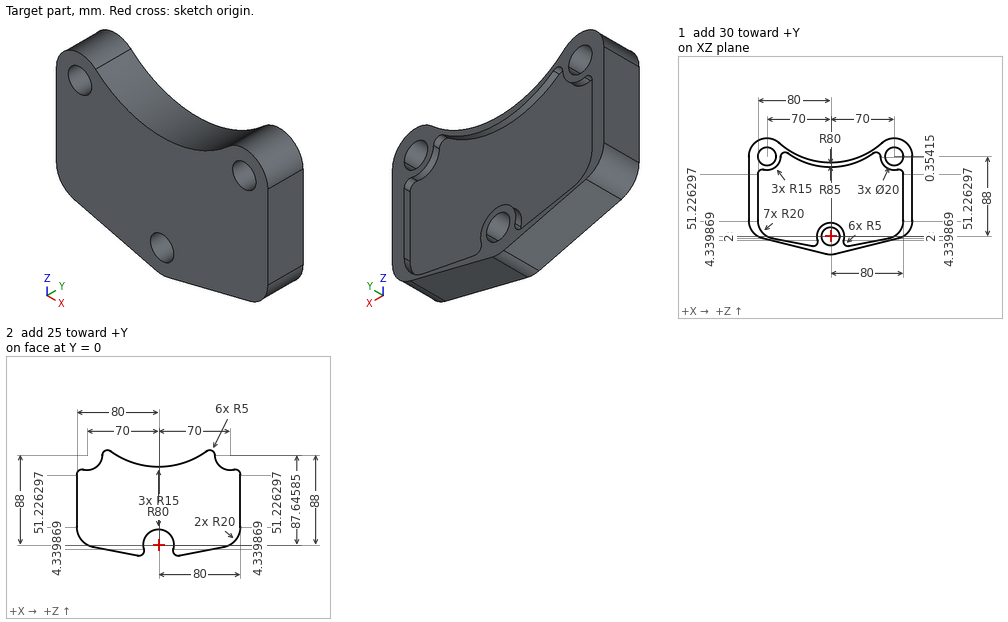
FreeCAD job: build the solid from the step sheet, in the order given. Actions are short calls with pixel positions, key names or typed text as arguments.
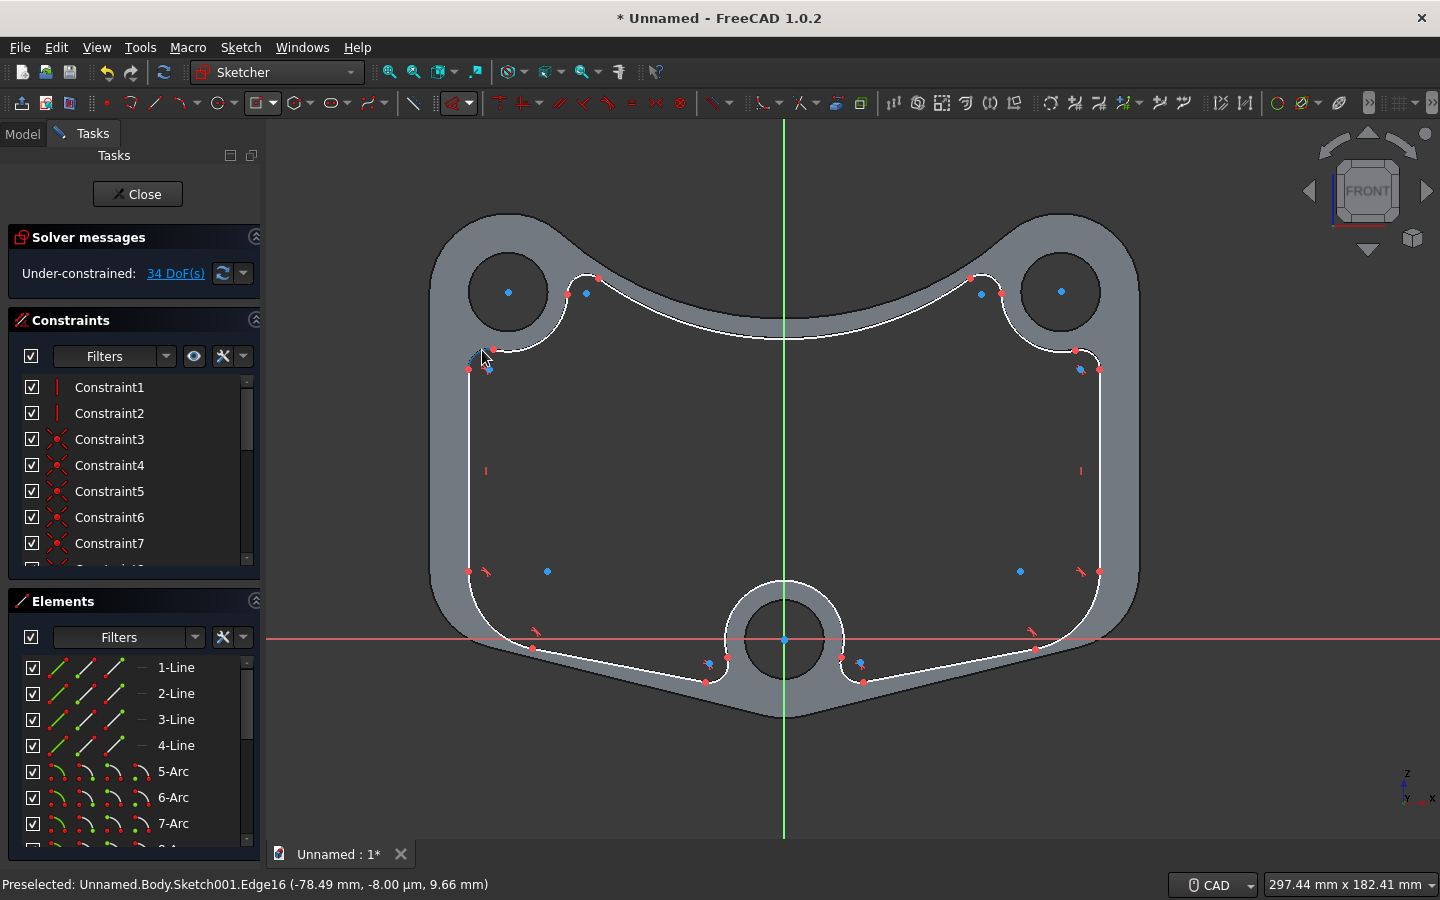
click(717, 681)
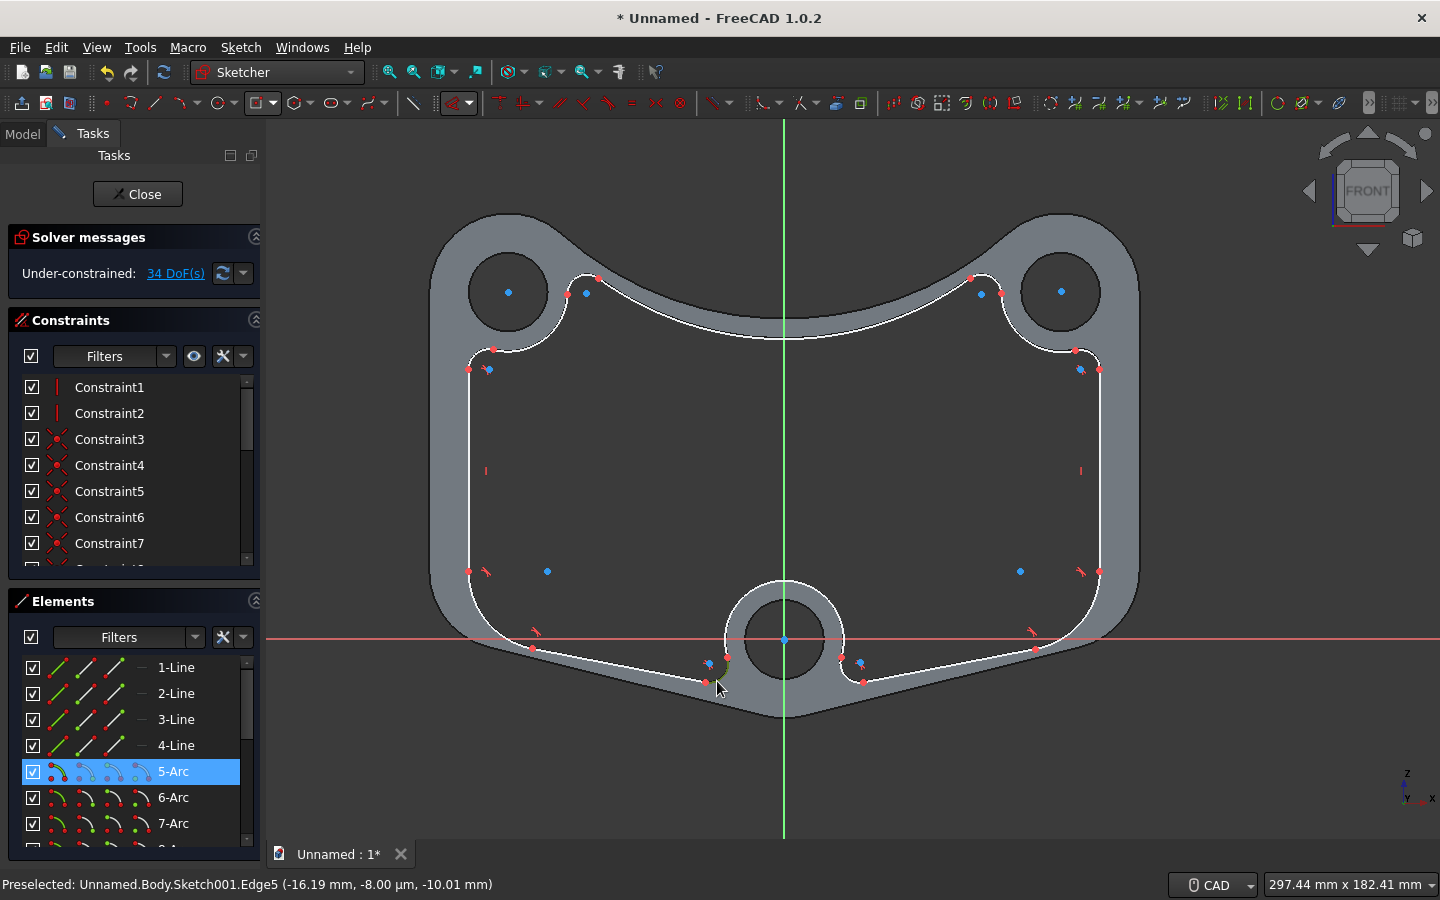
click(825, 596)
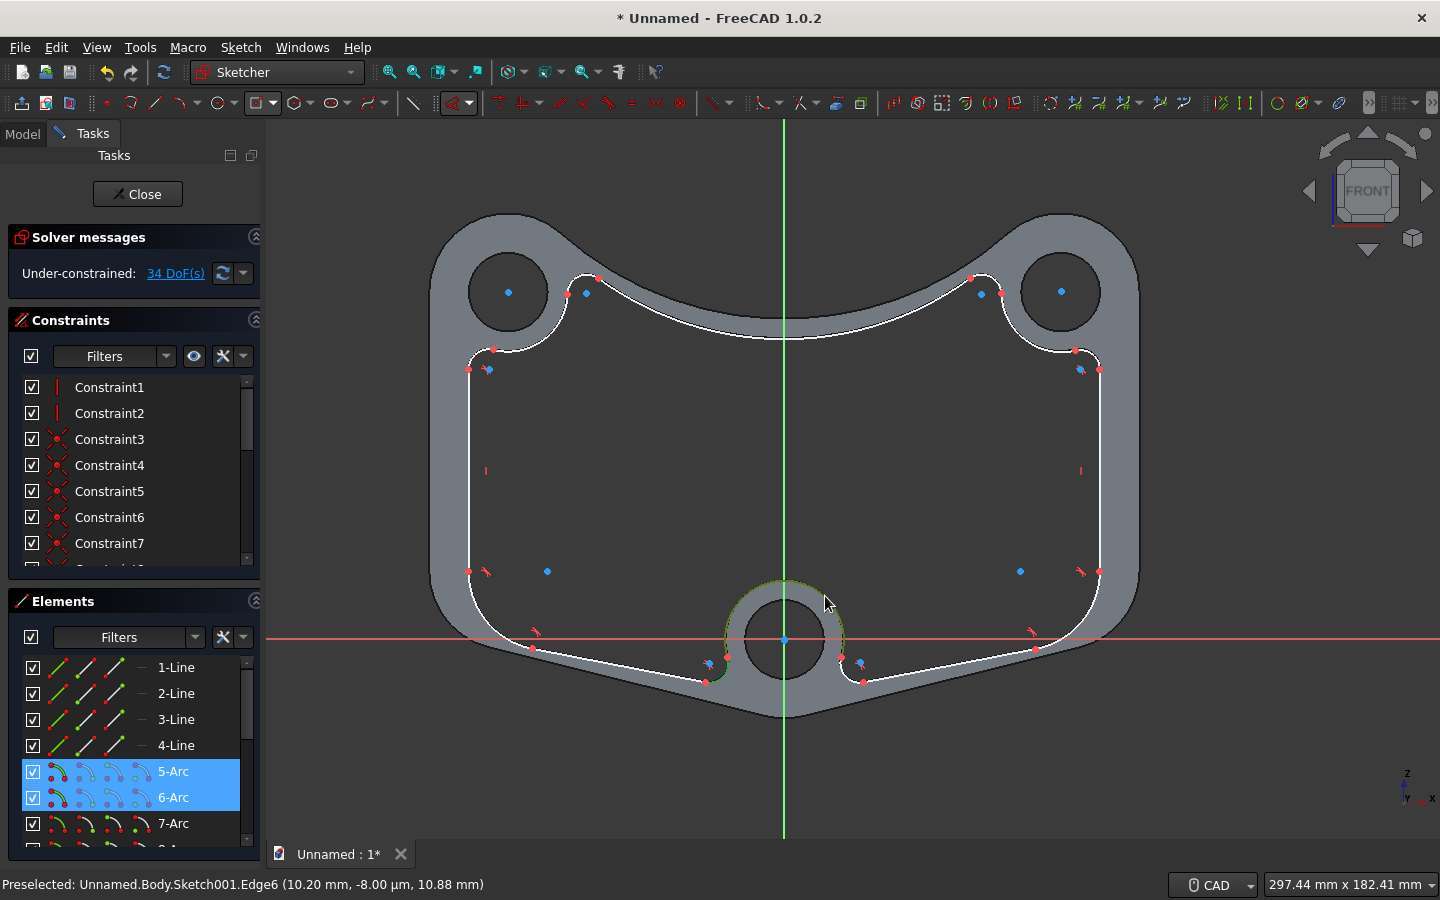
click(608, 104)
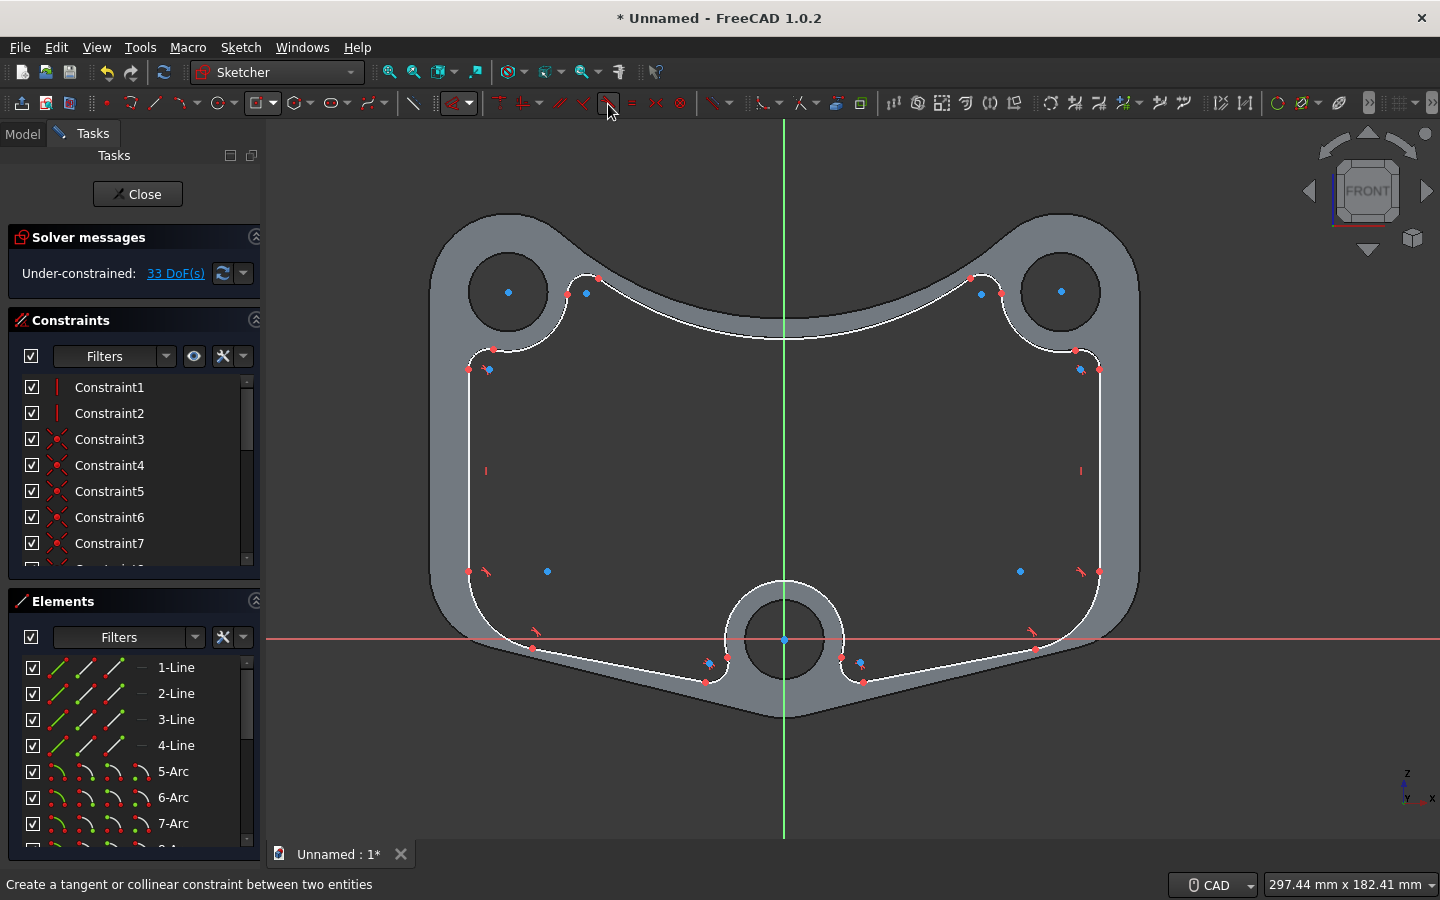
click(825, 597)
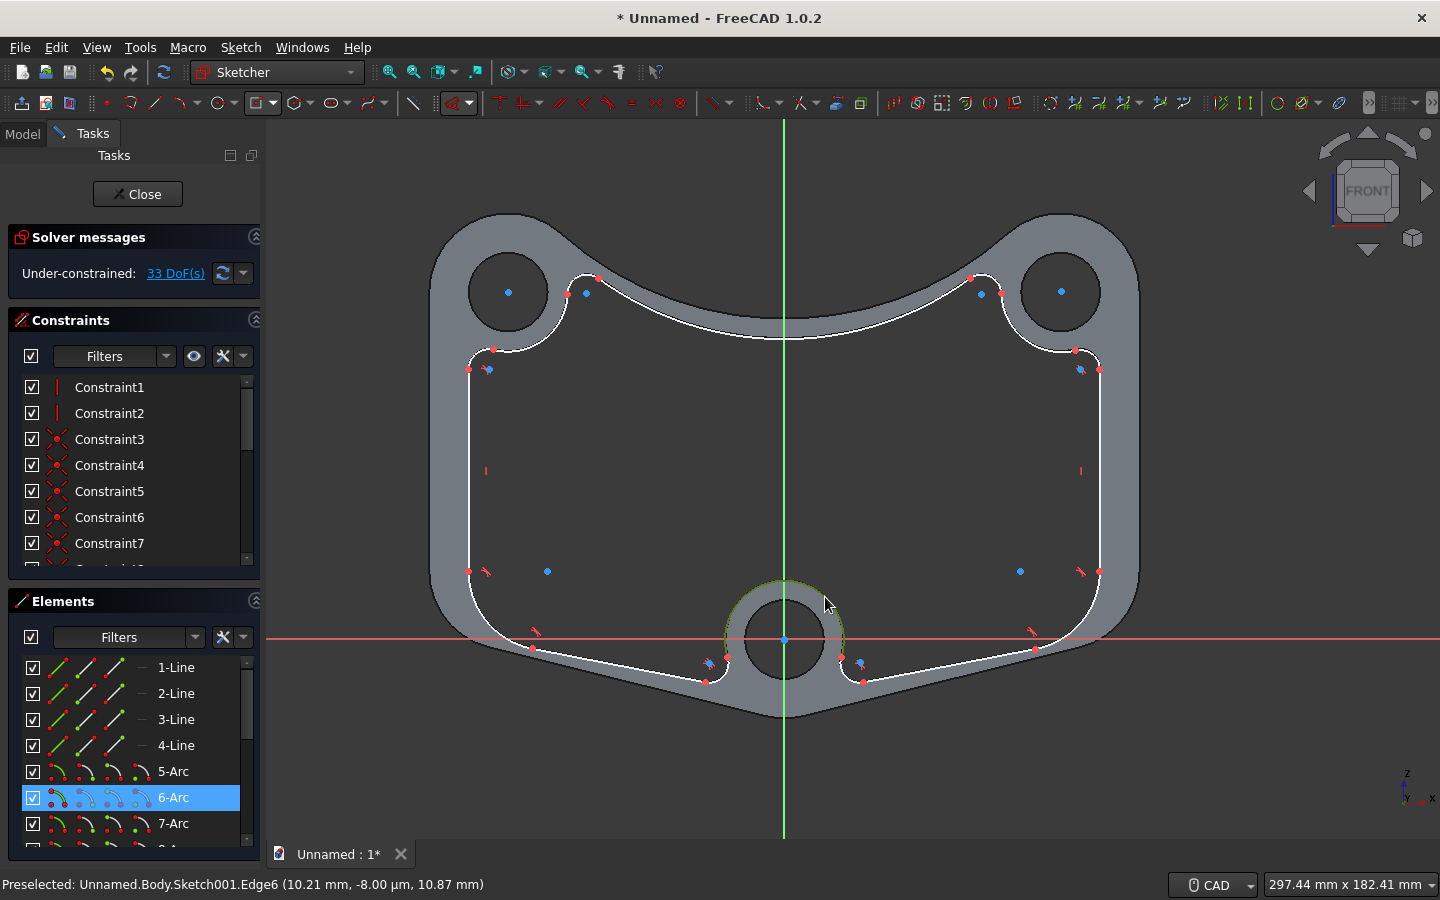
click(842, 669)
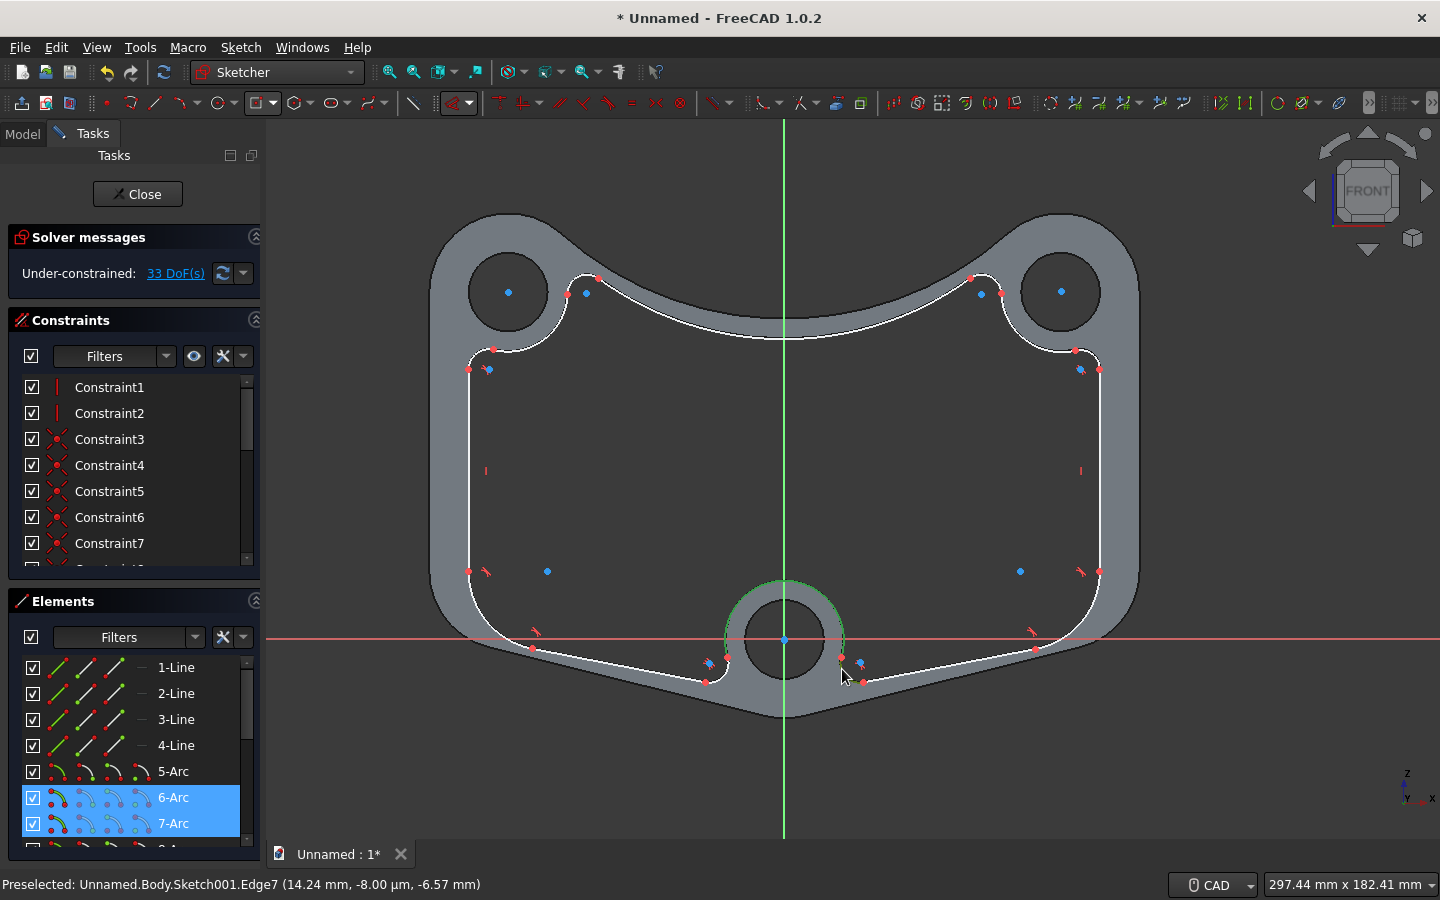
key(t)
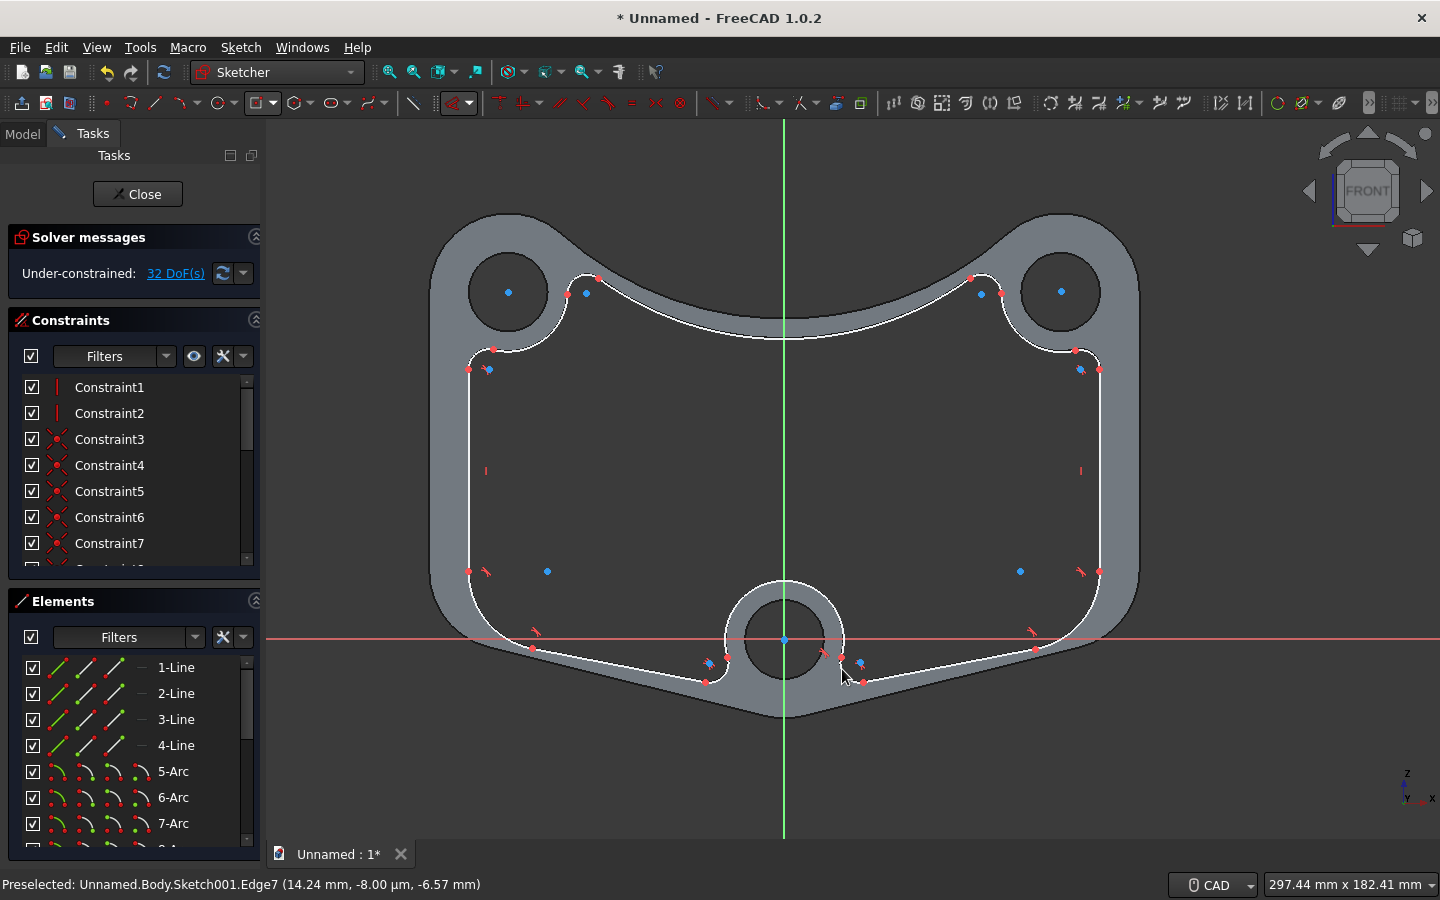
scroll(1097, 360, up, 2)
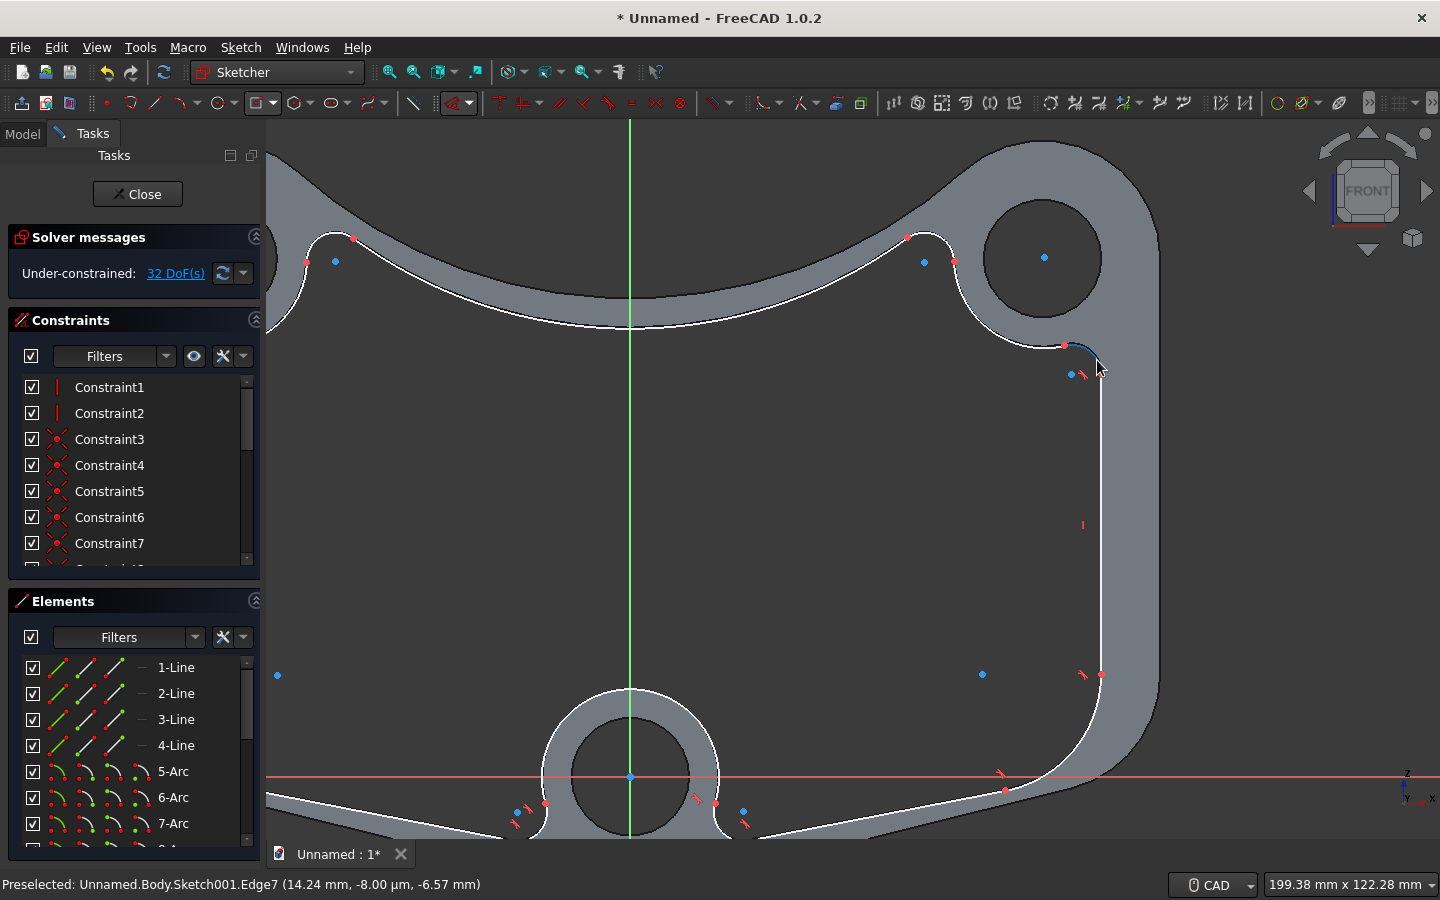
click(1097, 359)